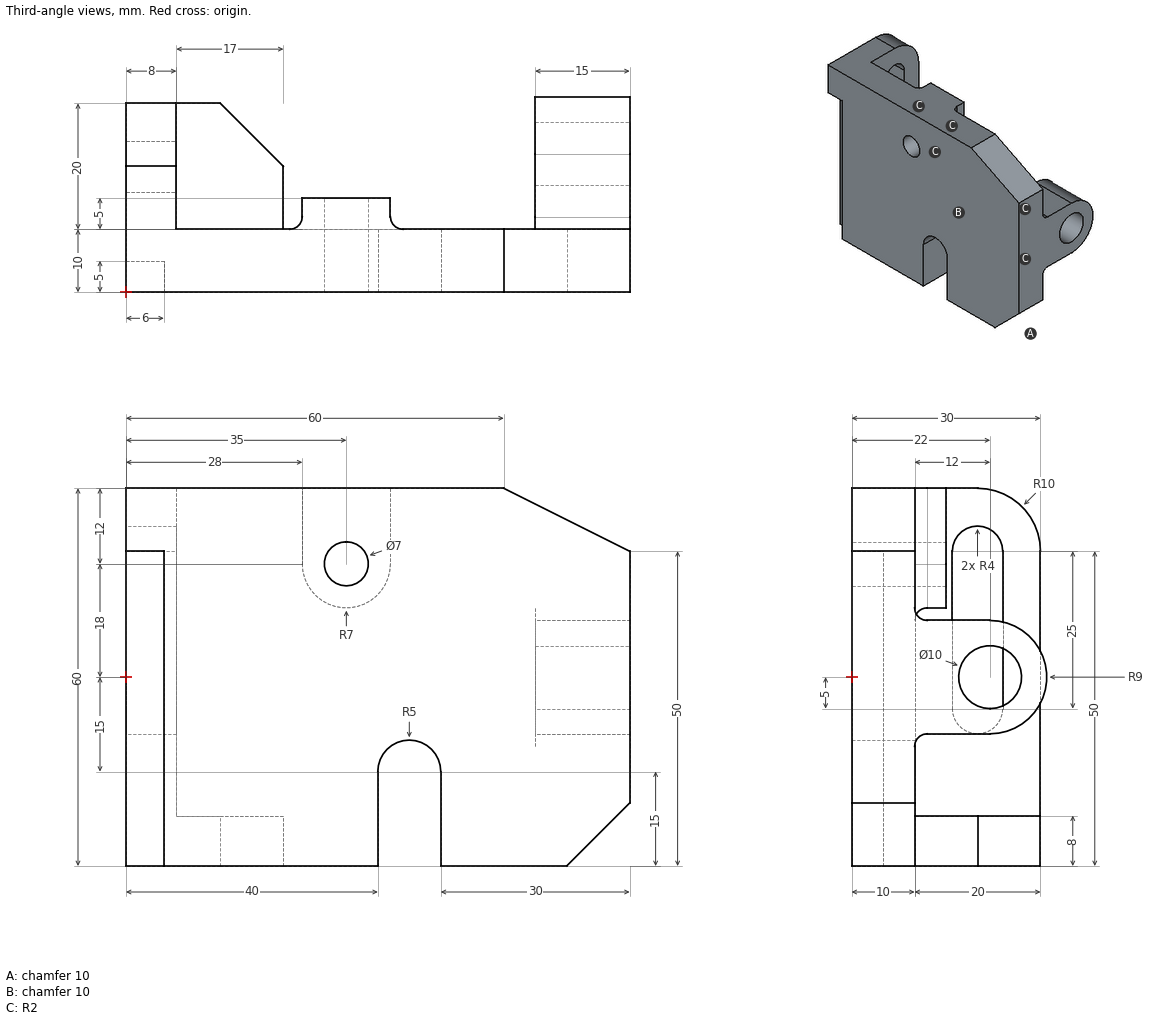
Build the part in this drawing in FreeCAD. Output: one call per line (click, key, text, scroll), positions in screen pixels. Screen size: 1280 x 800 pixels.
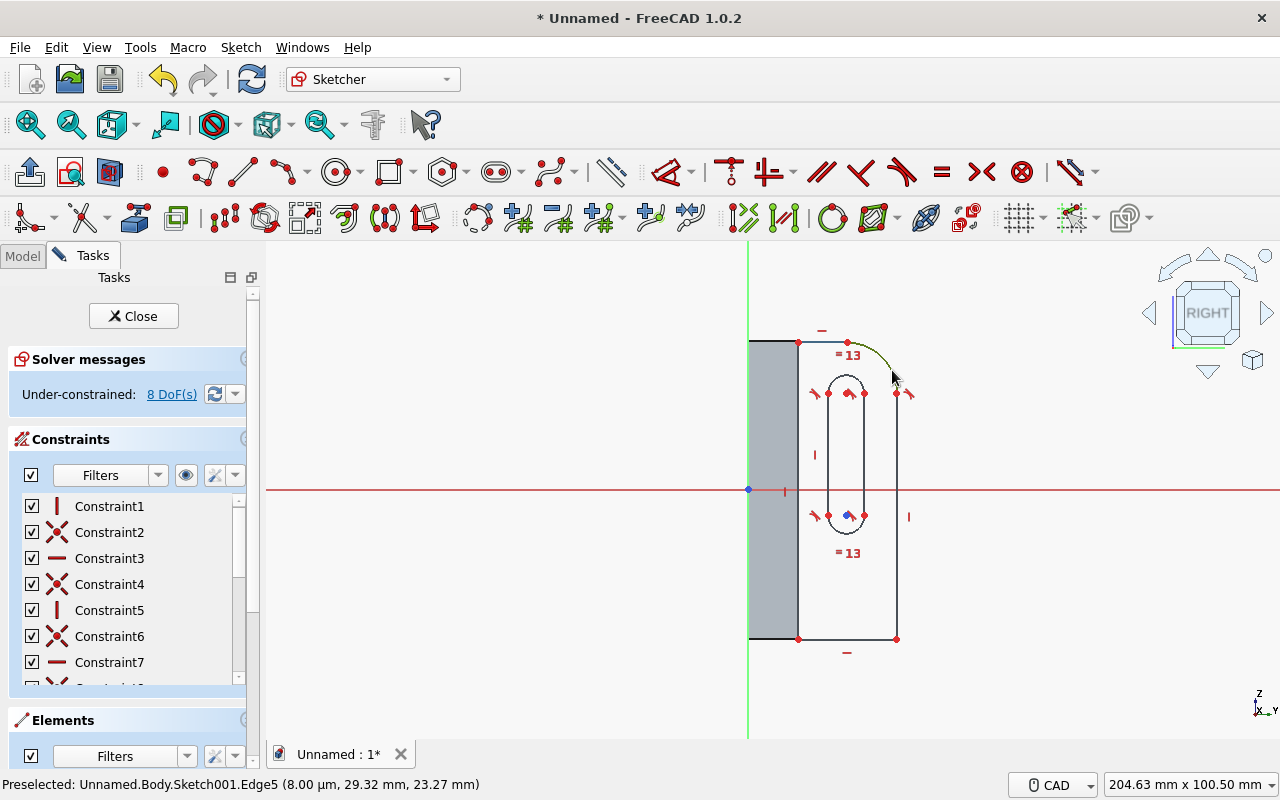
click(902, 172)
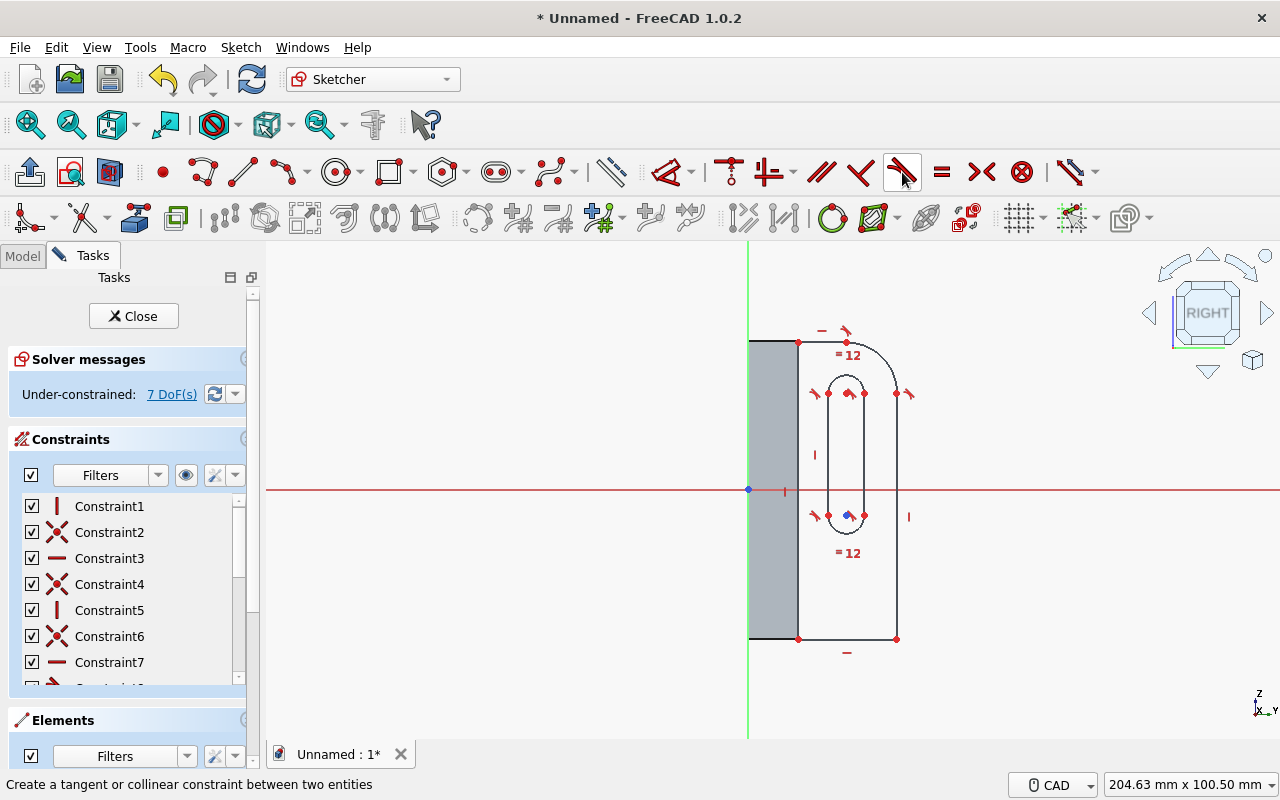
key(d)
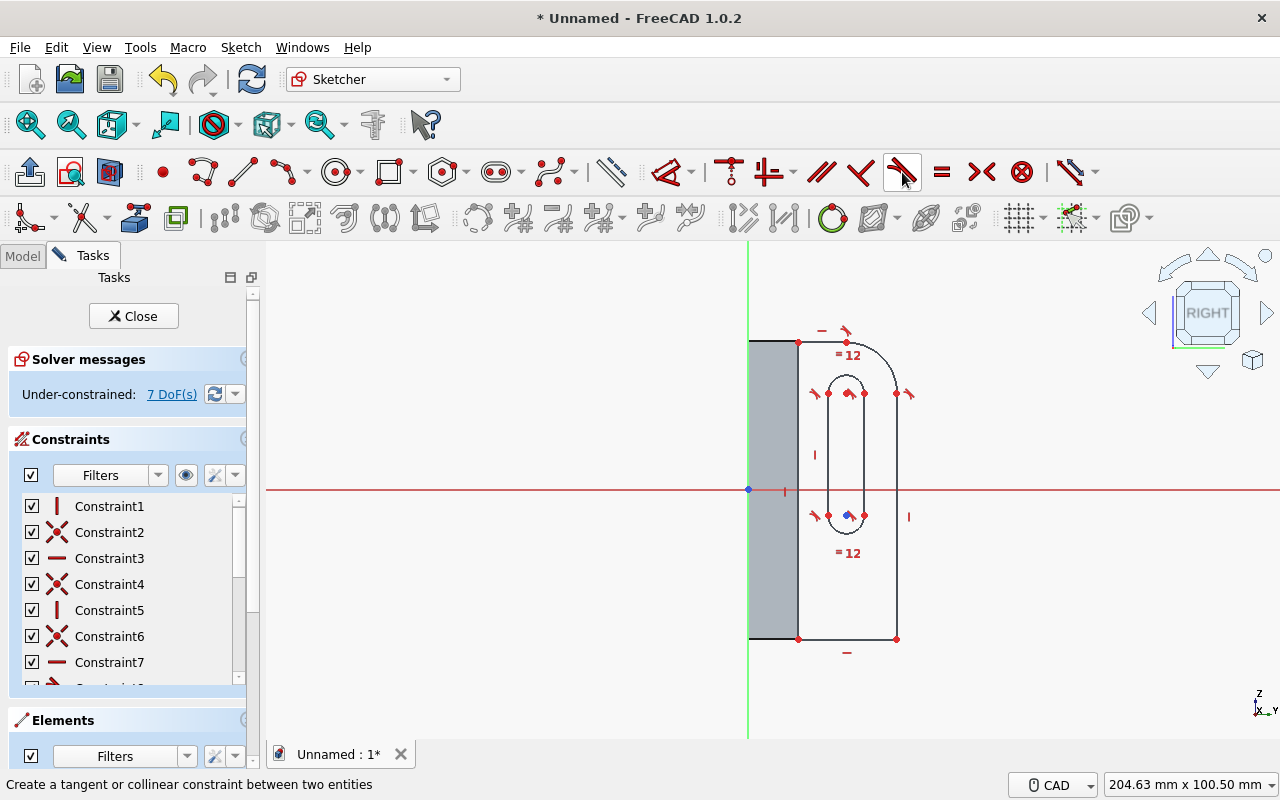
click(891, 370)
click(919, 355)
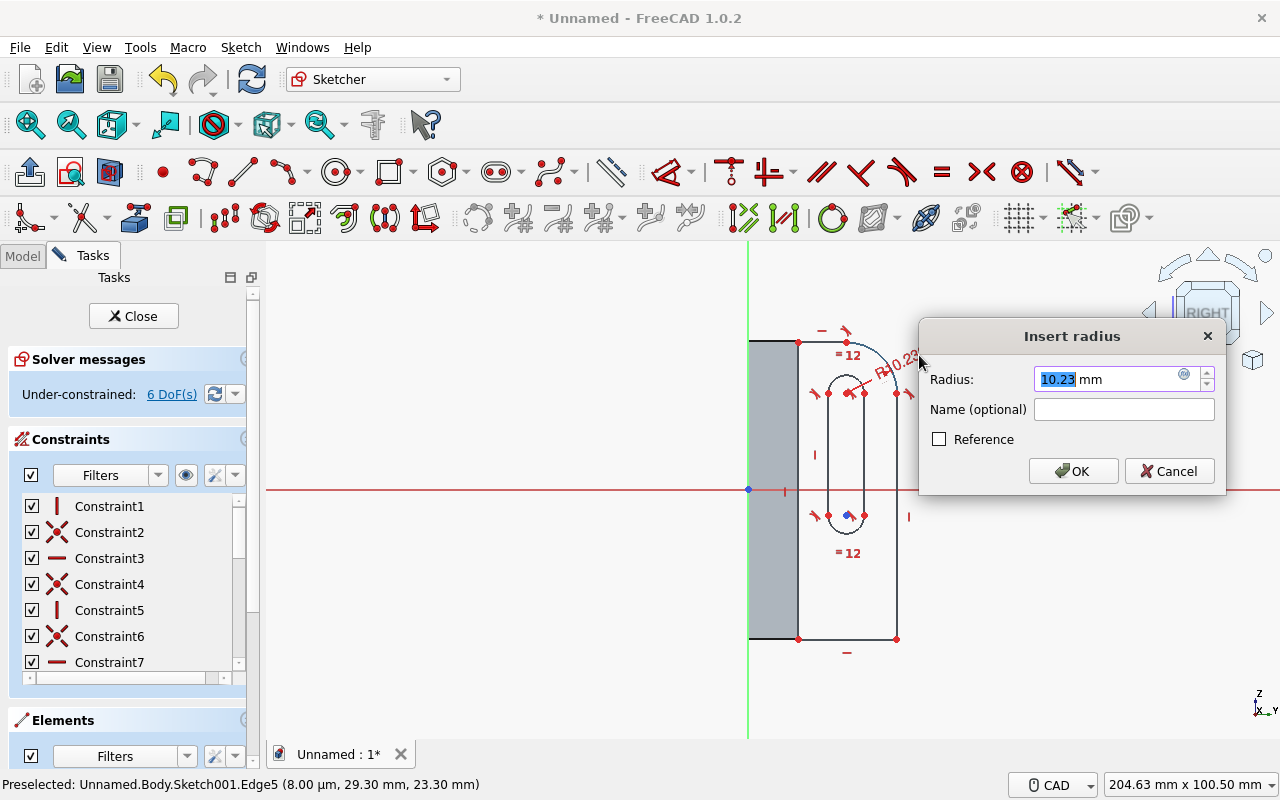
text(10)
key(Return)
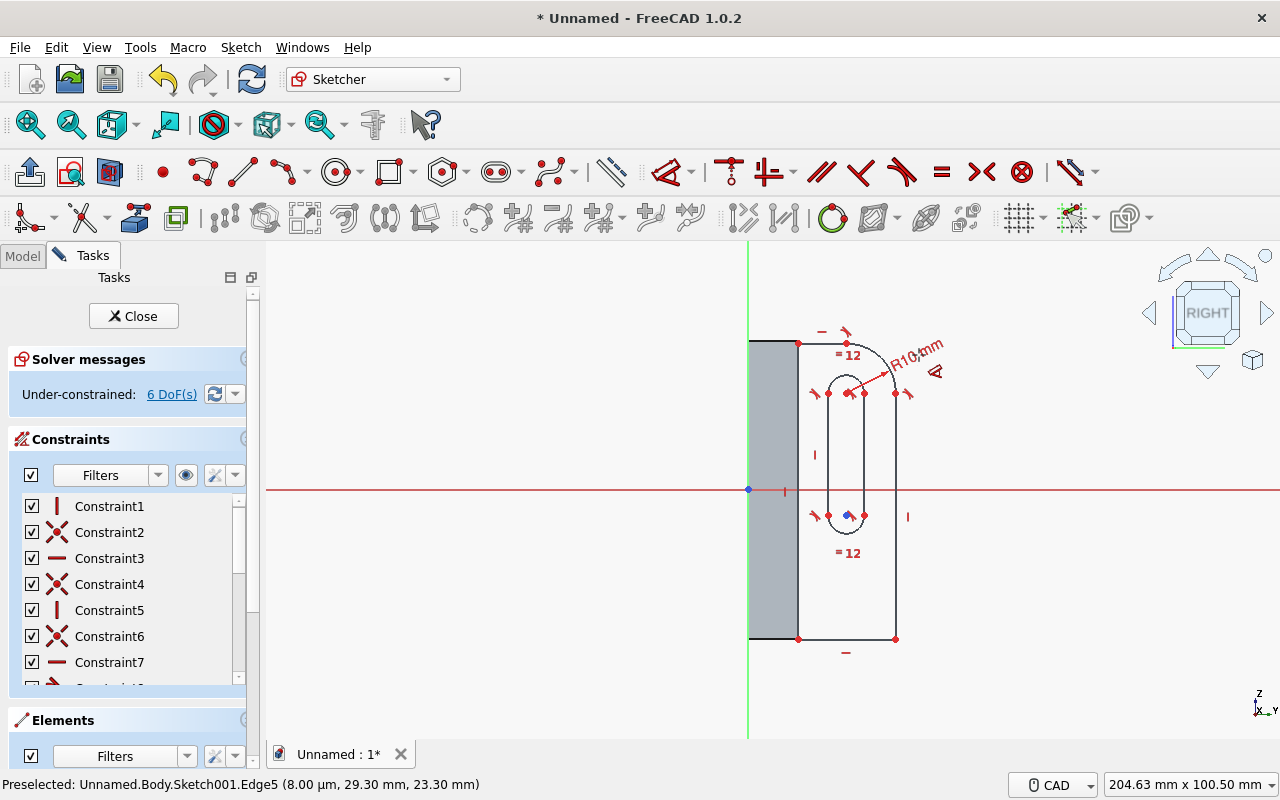
scroll(836, 530, up, 4)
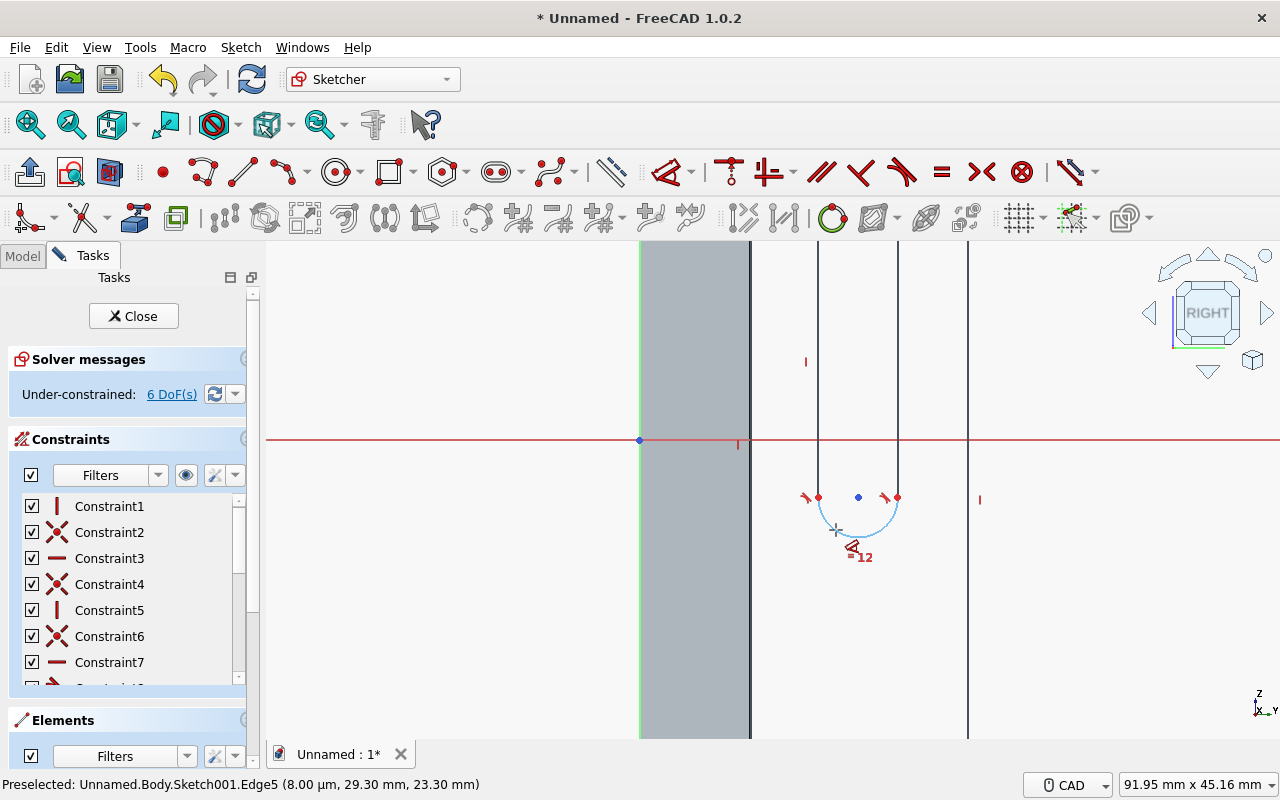
click(835, 530)
click(816, 556)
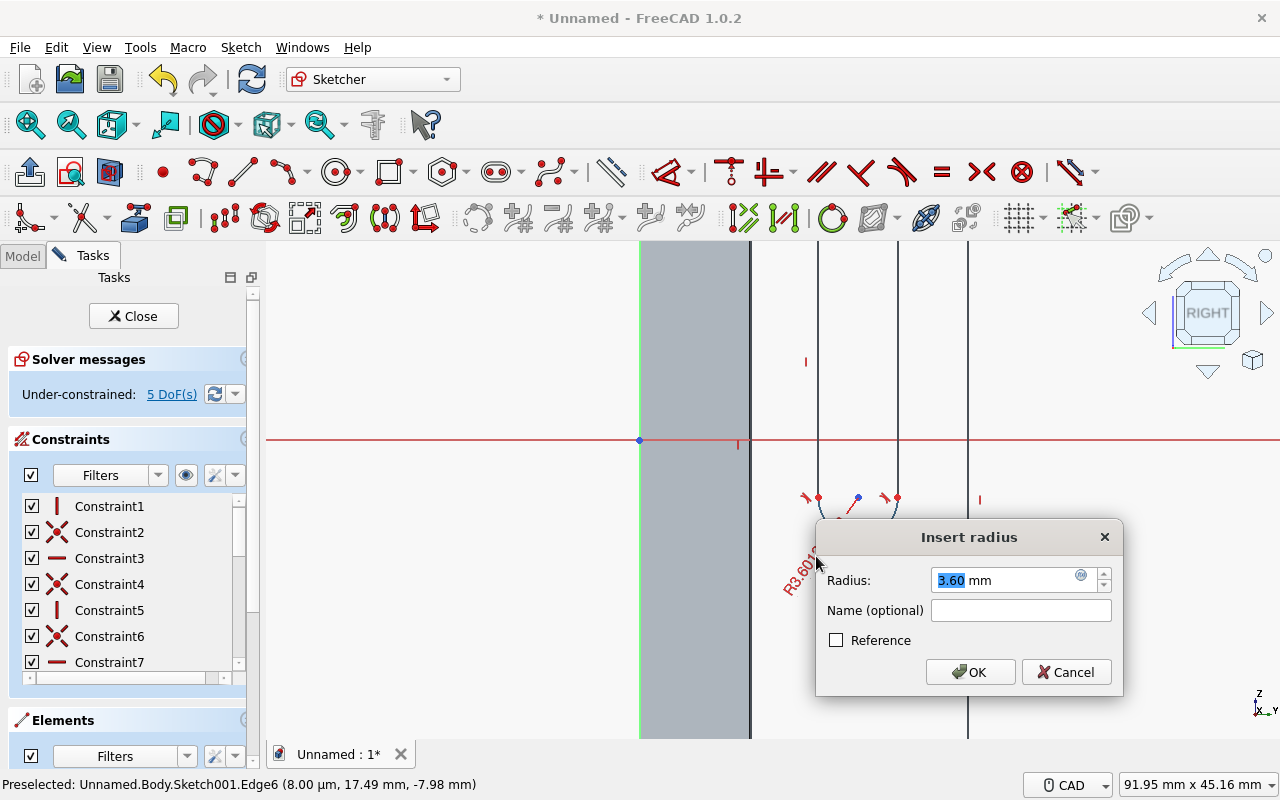
text(4)
key(Return)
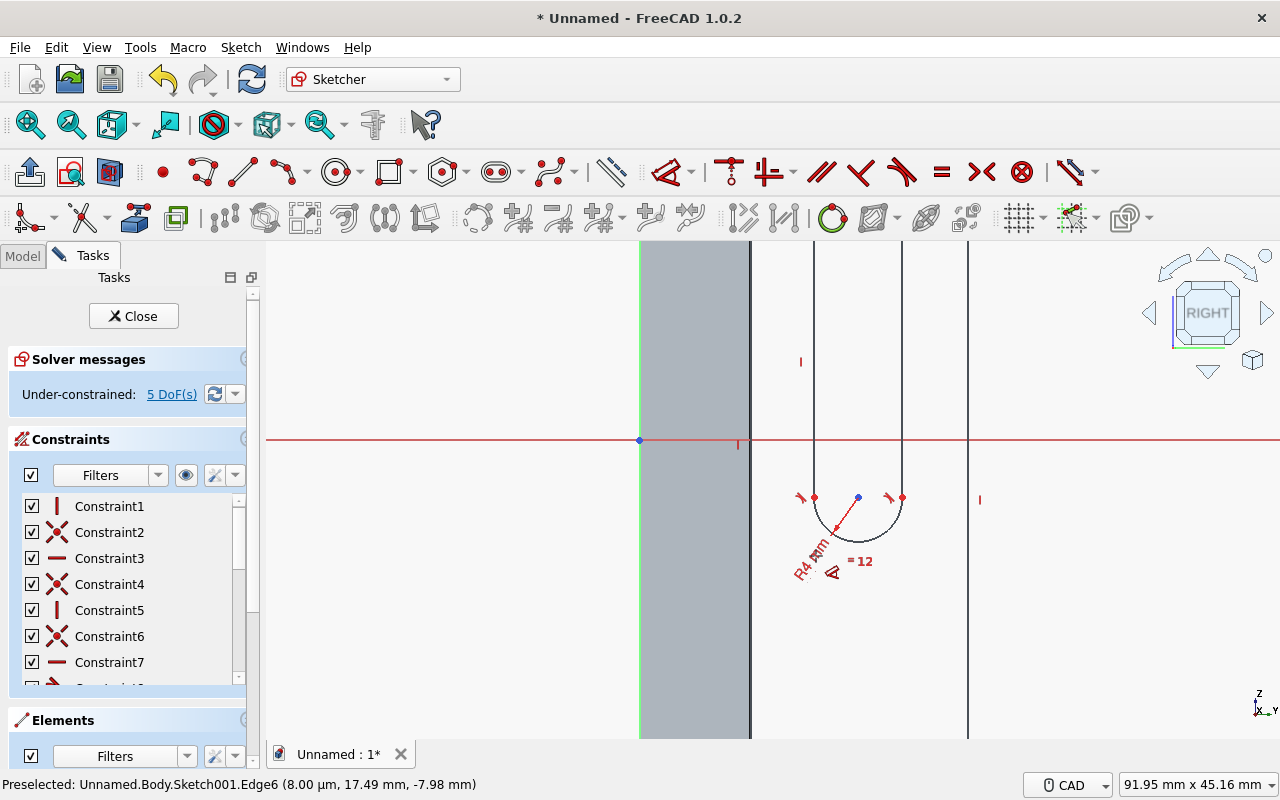
click(968, 390)
click(1002, 490)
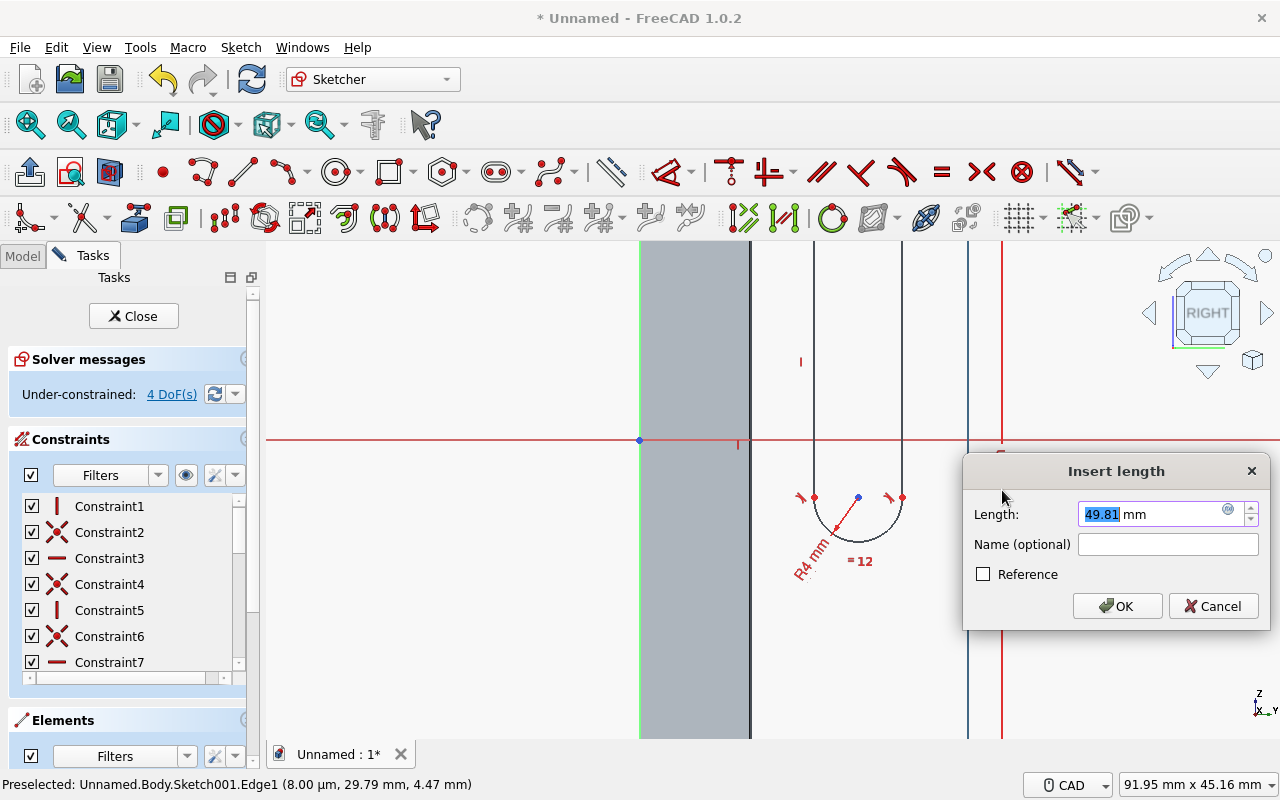
text(50)
key(Return)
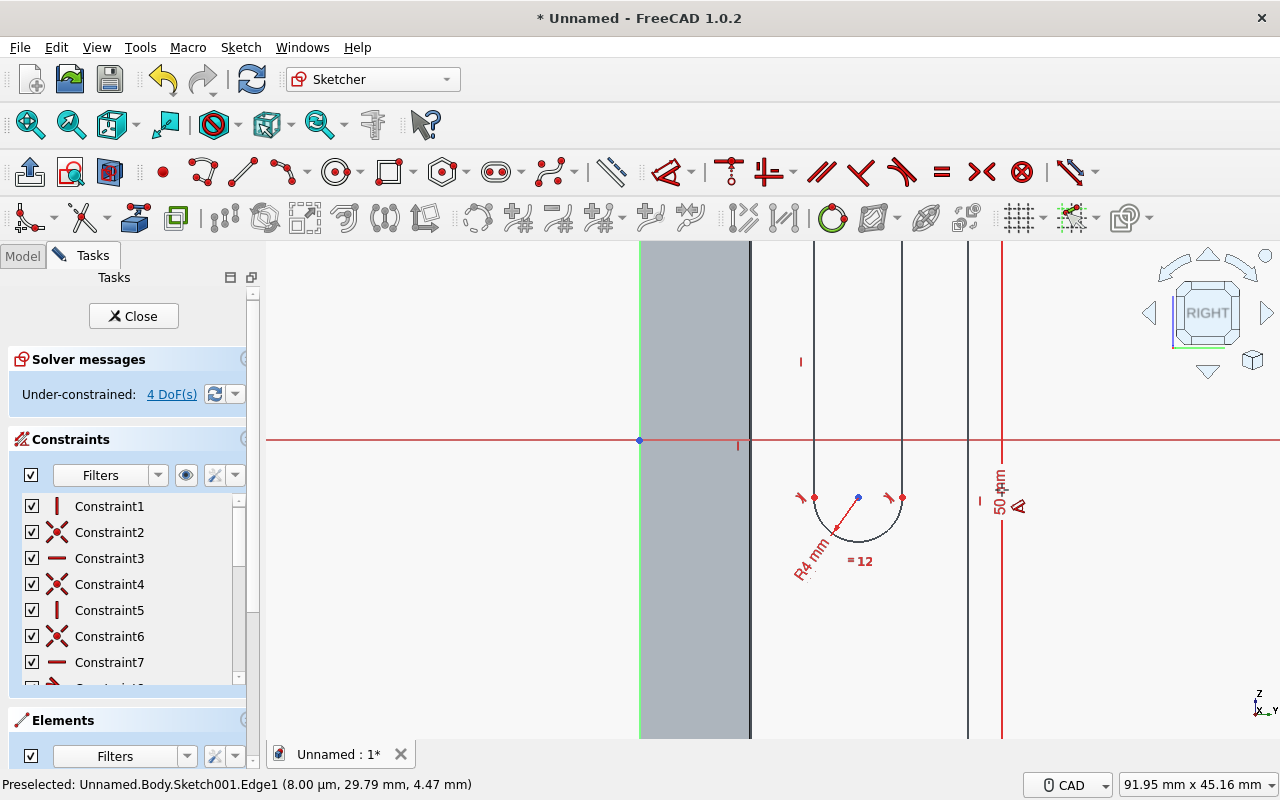
scroll(622, 531, down, 4)